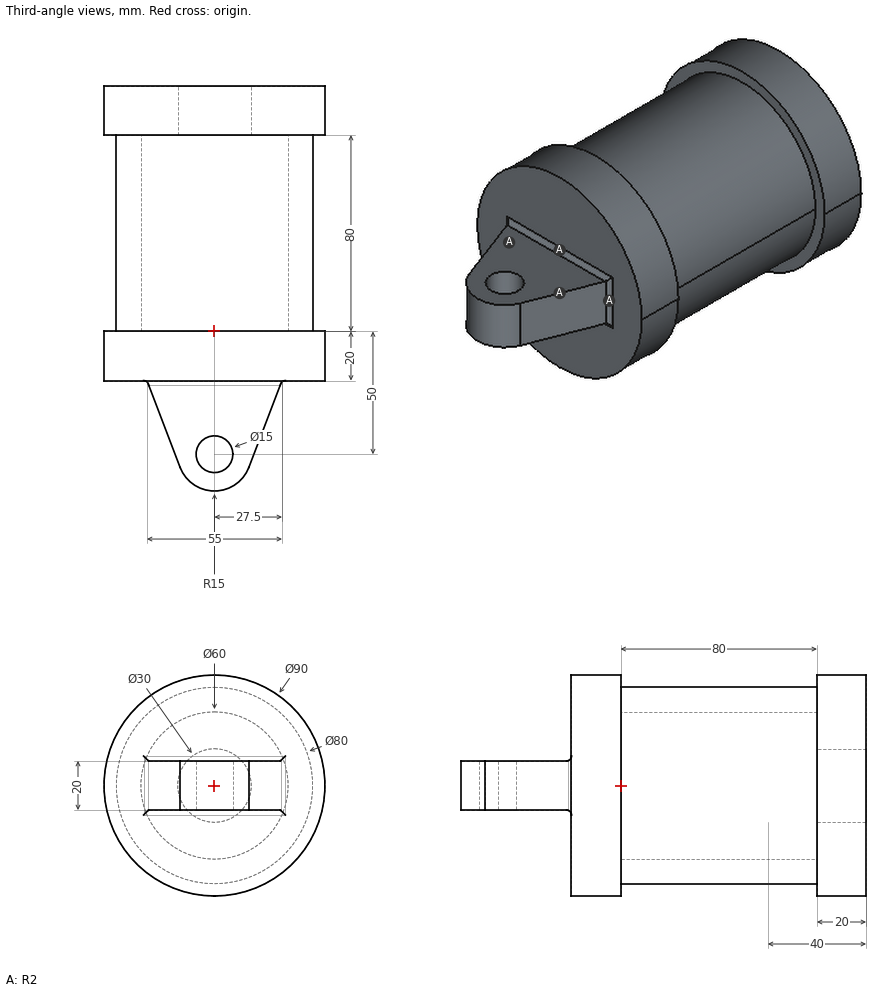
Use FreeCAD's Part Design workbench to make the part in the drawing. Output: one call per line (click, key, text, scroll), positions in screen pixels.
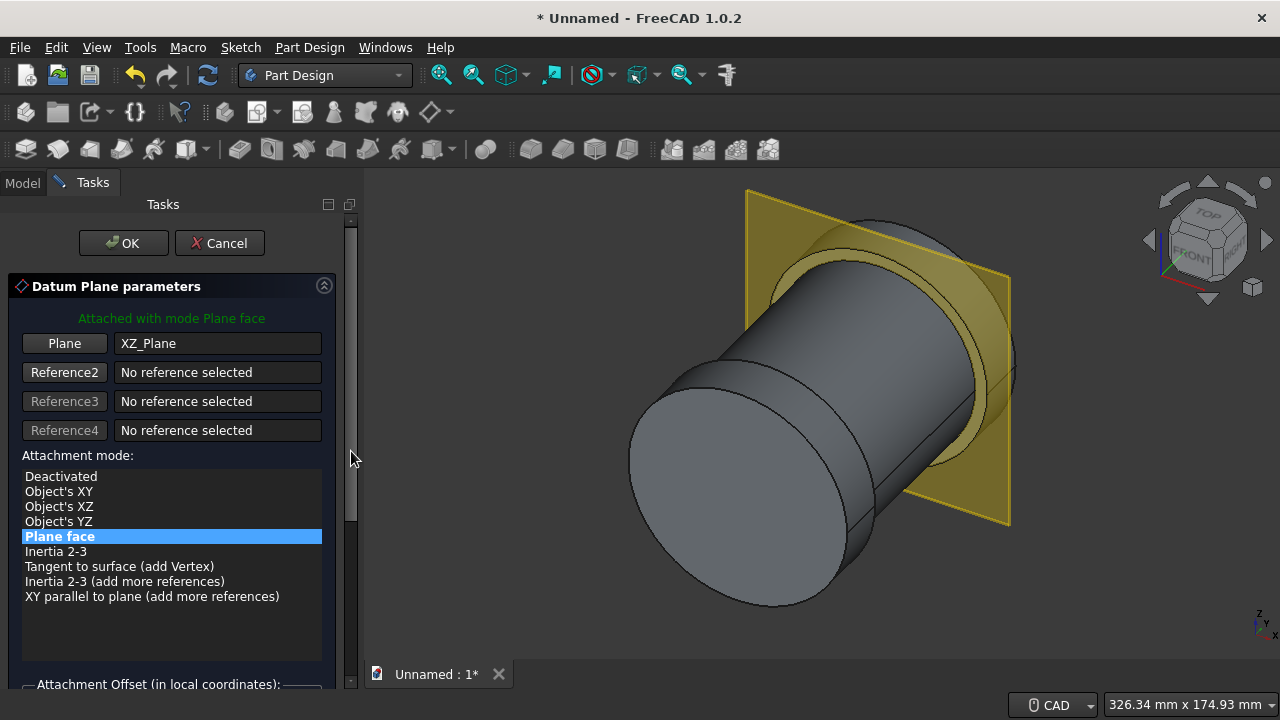
click(124, 243)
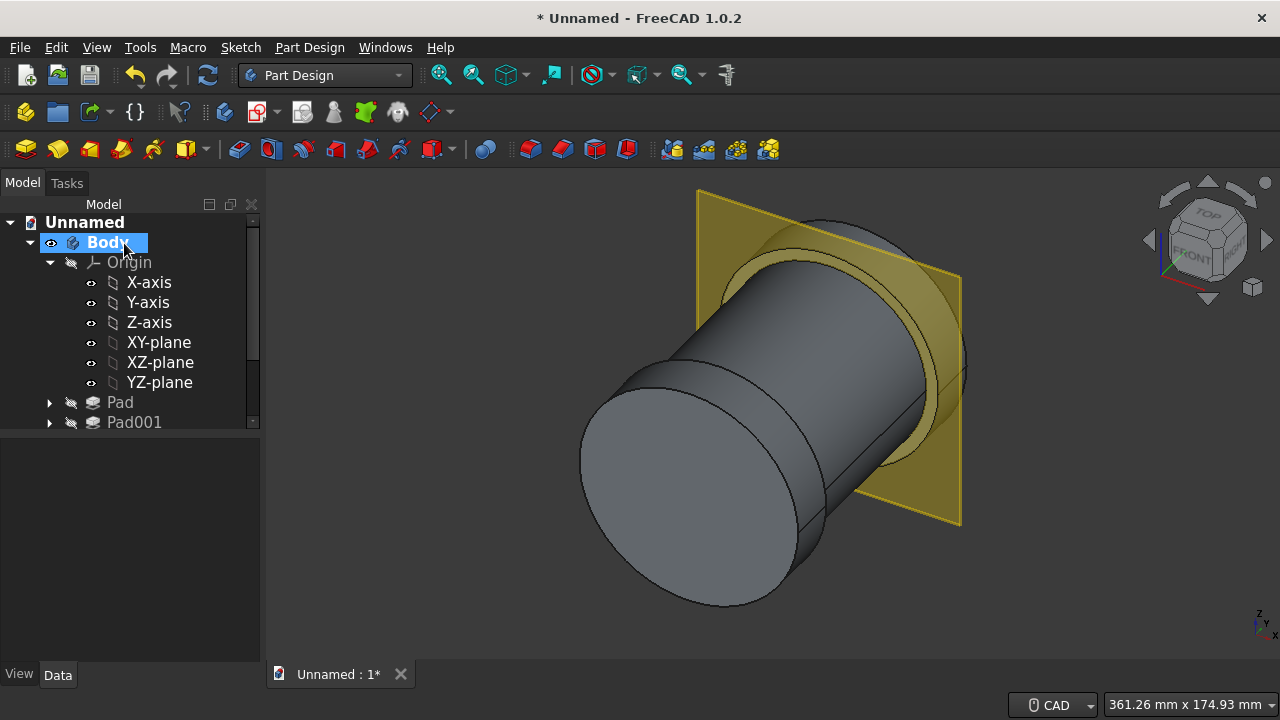
scroll(100, 318, down, 3)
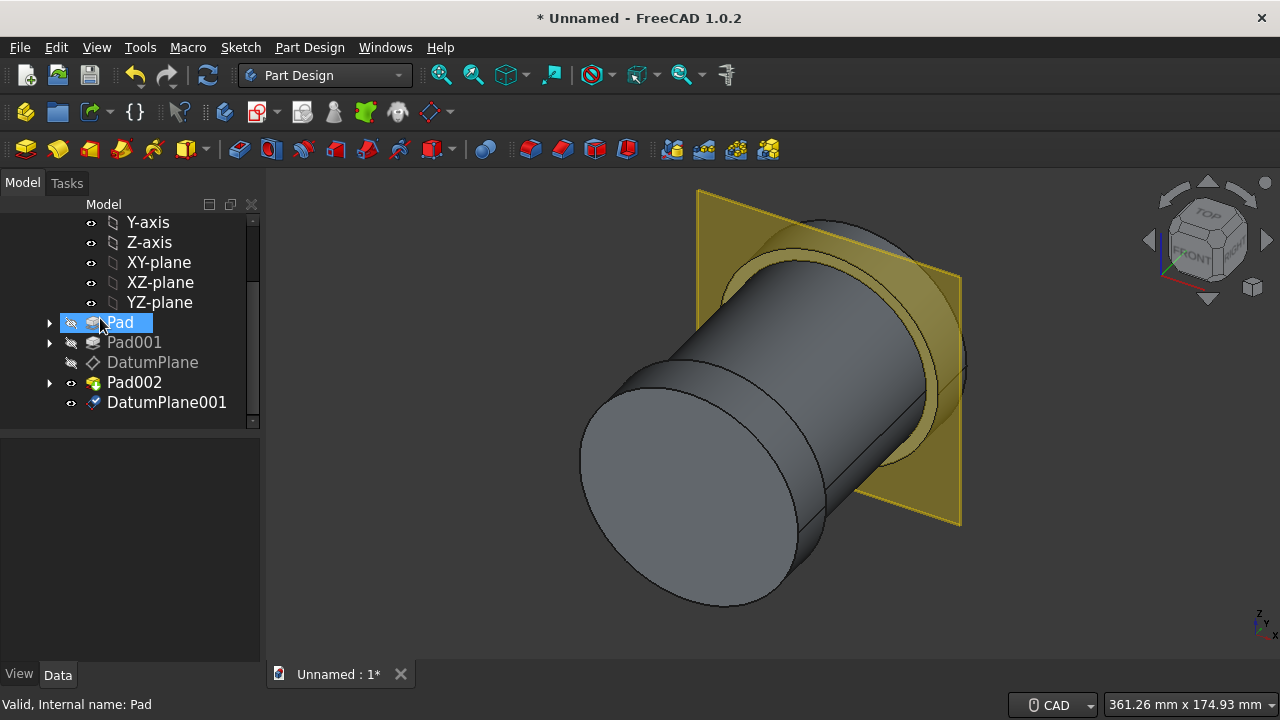
click(116, 403)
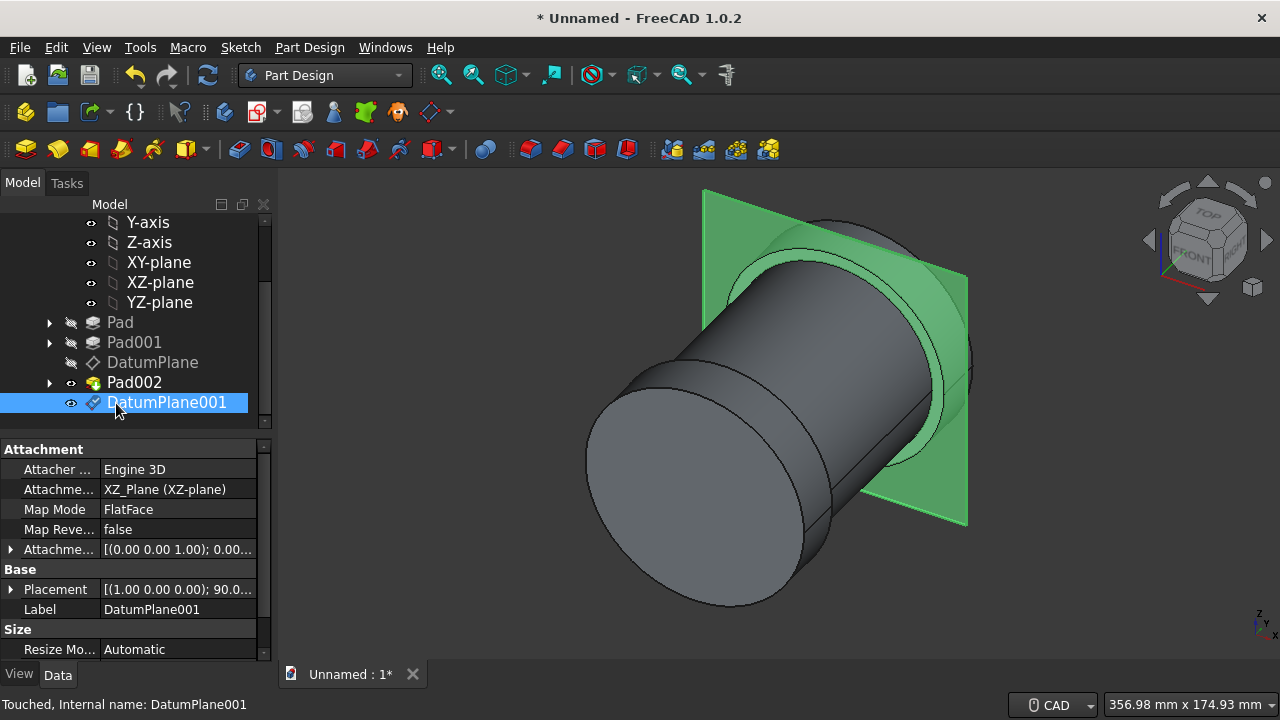
click(258, 112)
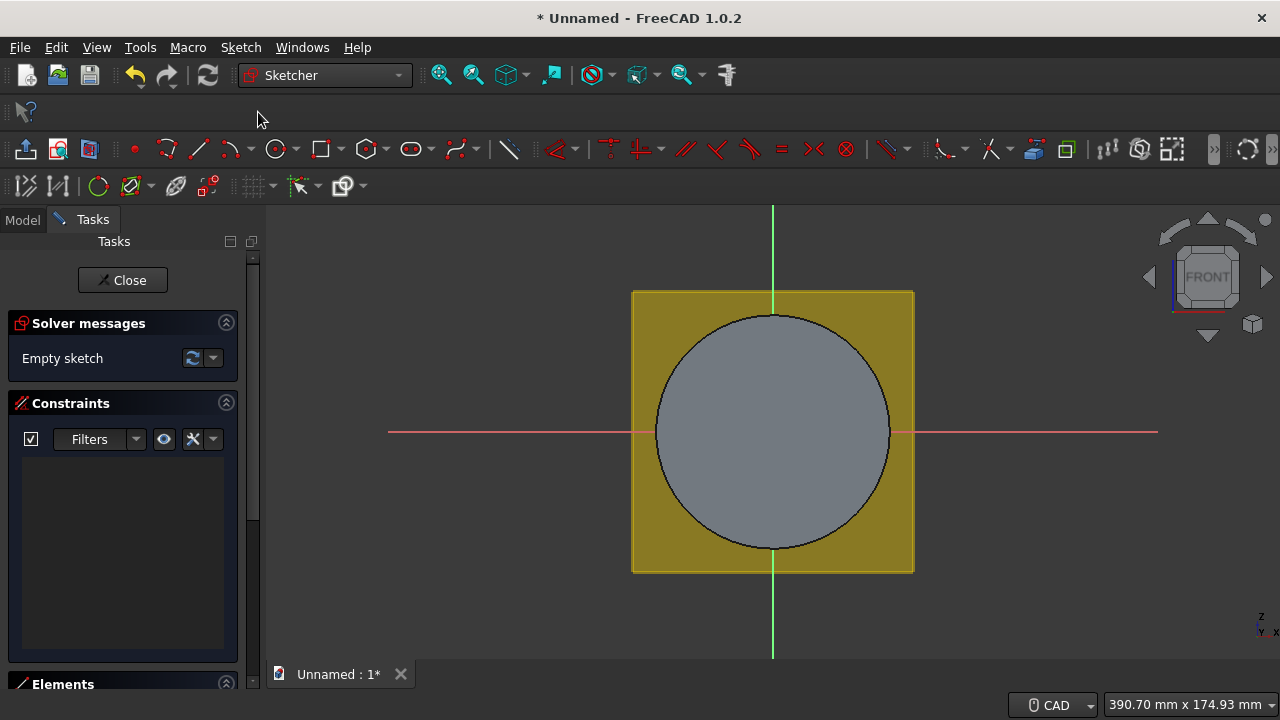
click(90, 150)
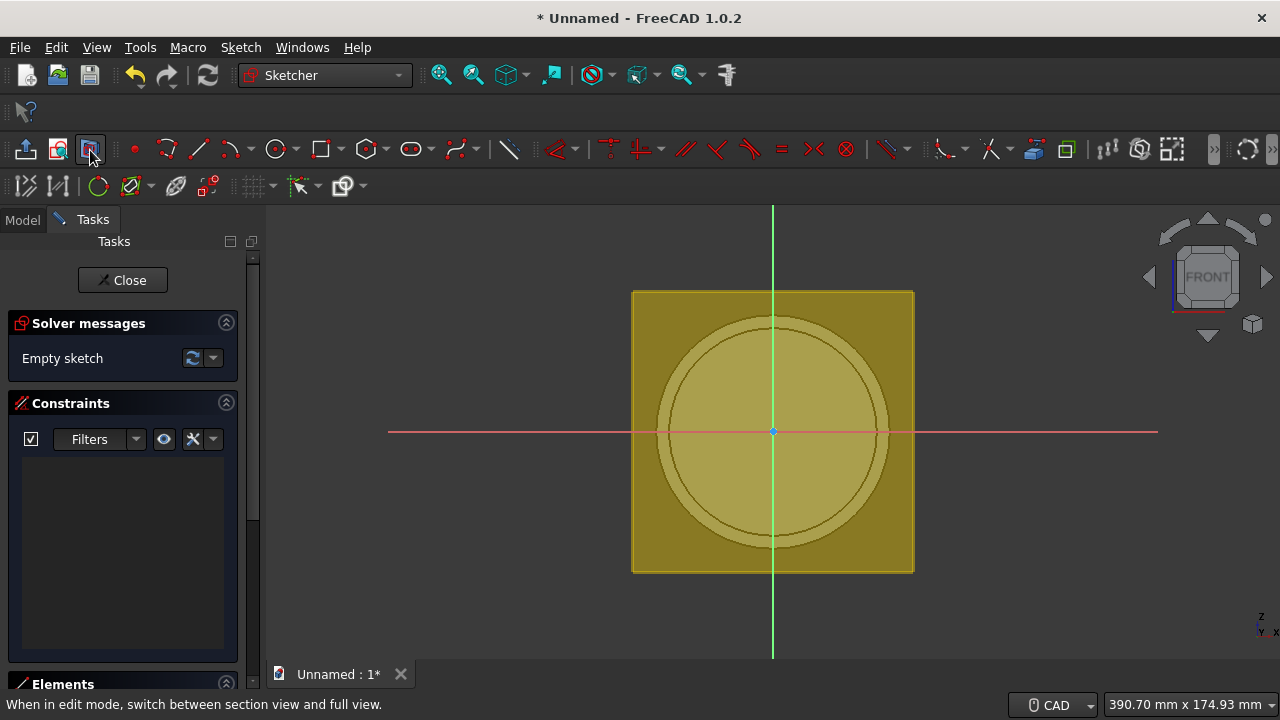
scroll(856, 432, up, 3)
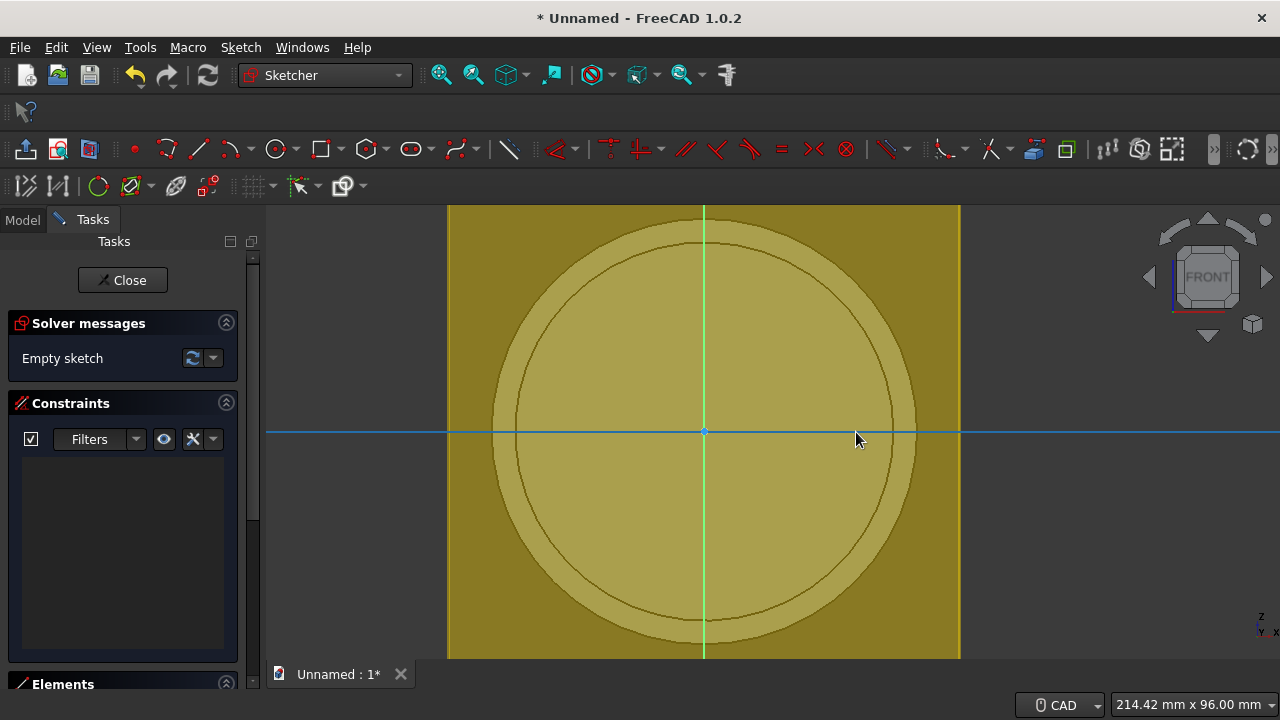
key(g)
key(c)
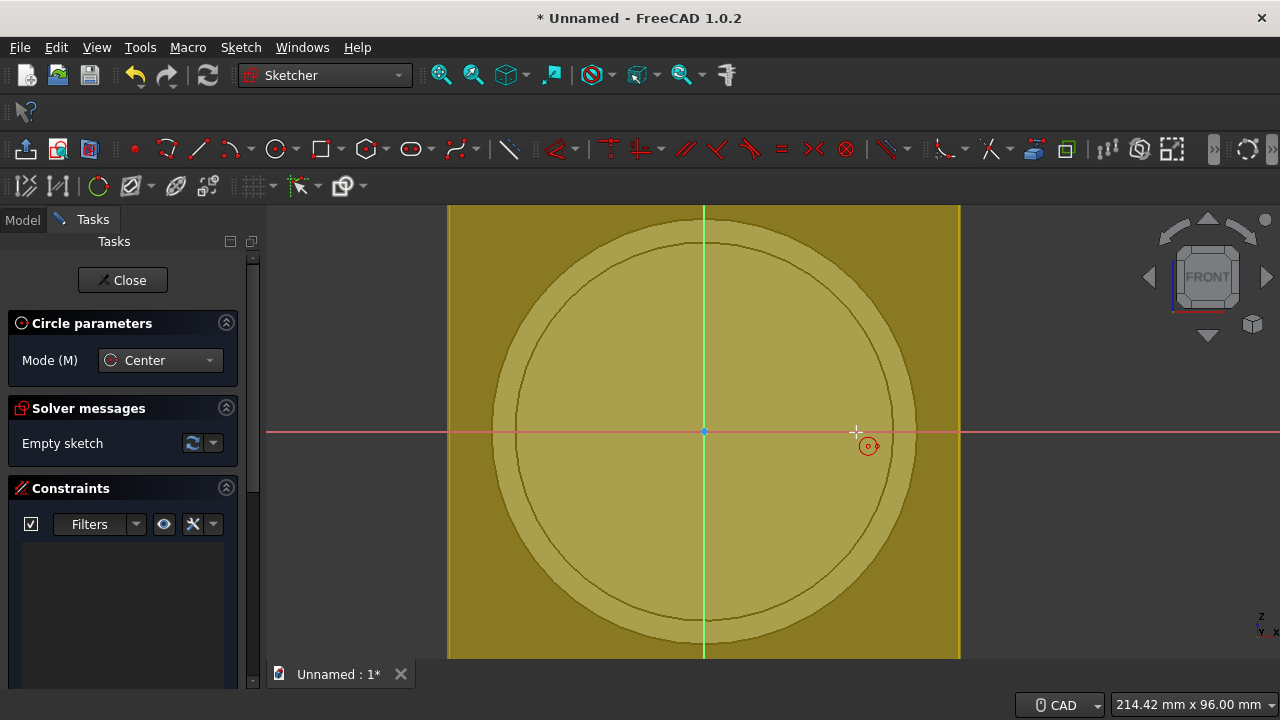
click(704, 432)
move(805, 331)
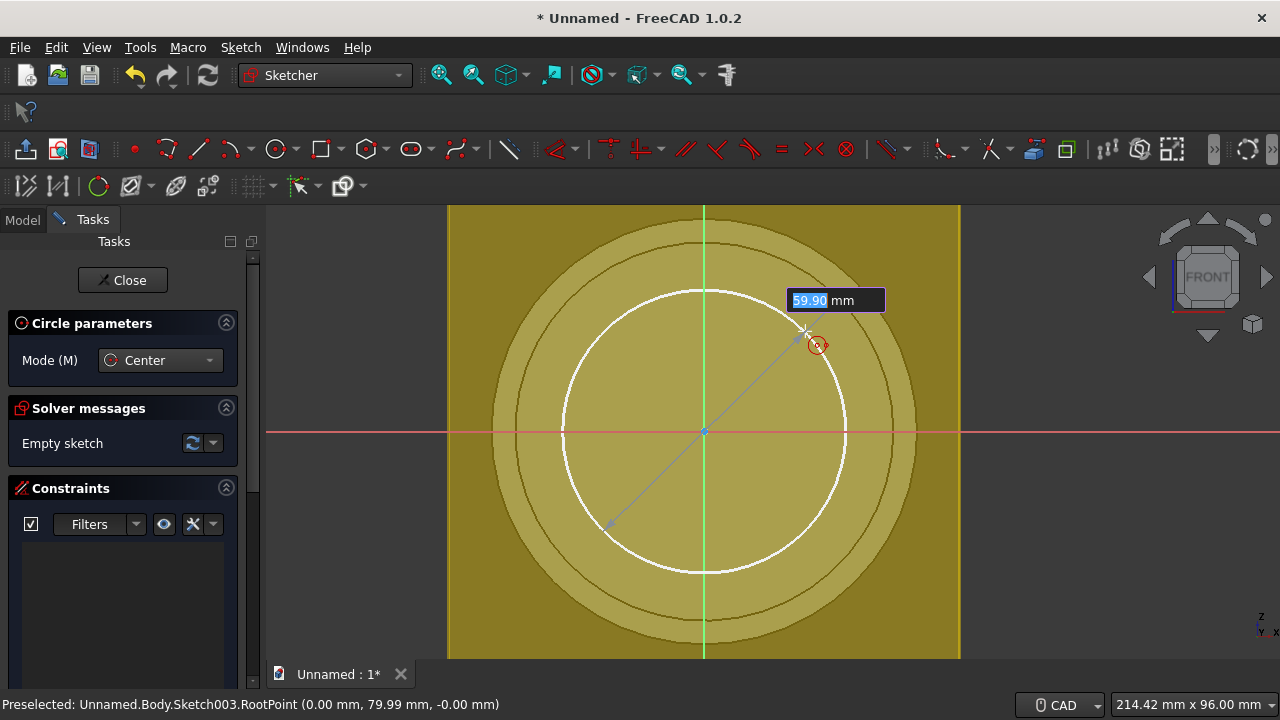
text(60)
key(Return)
key(Escape)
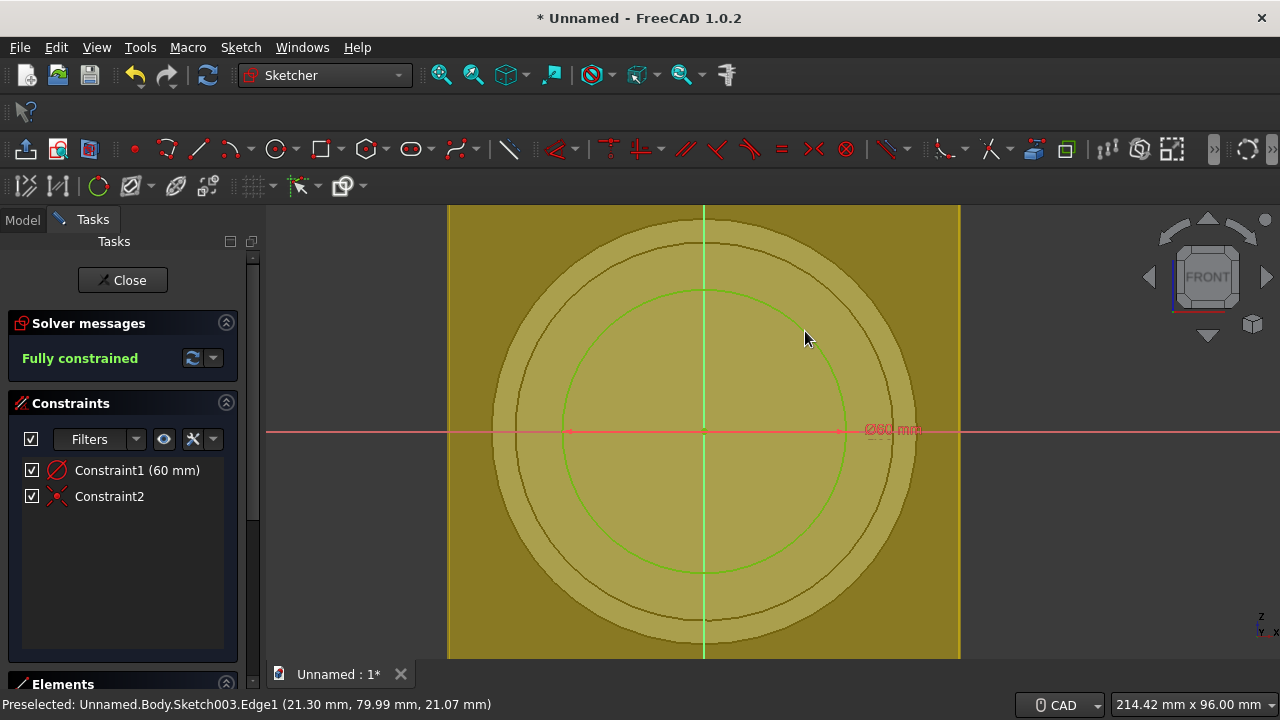
click(123, 280)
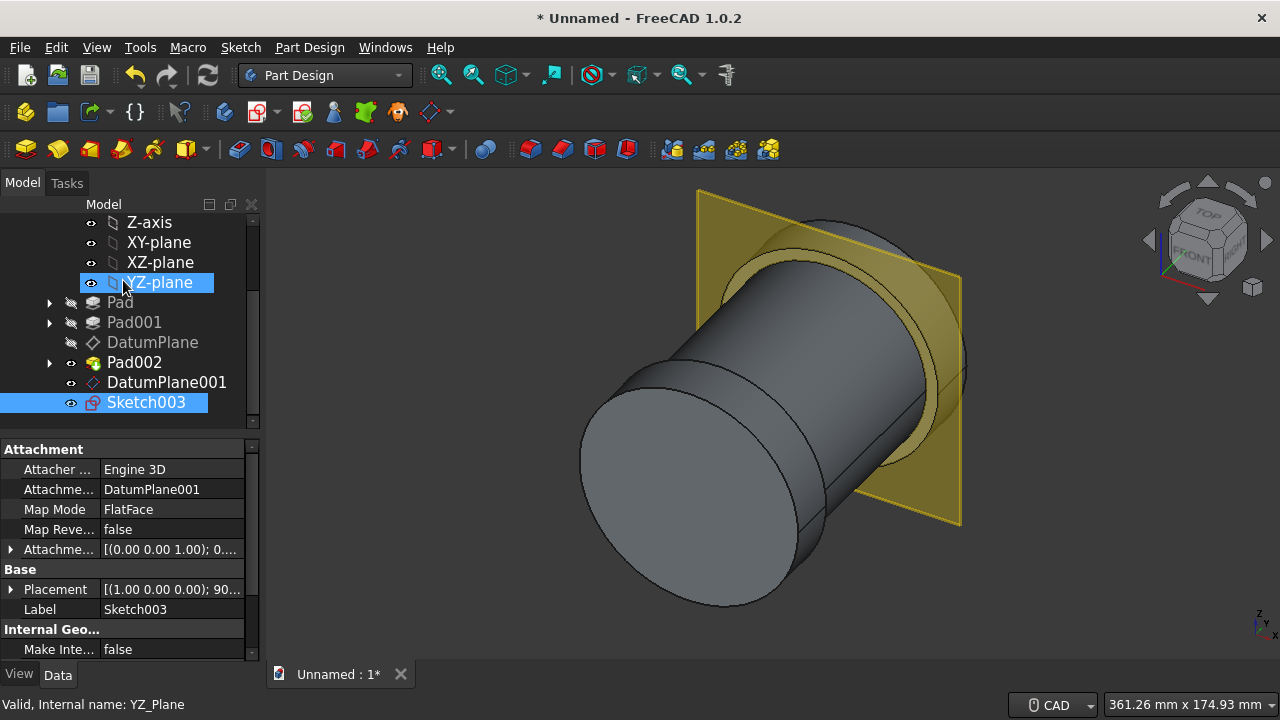
click(240, 150)